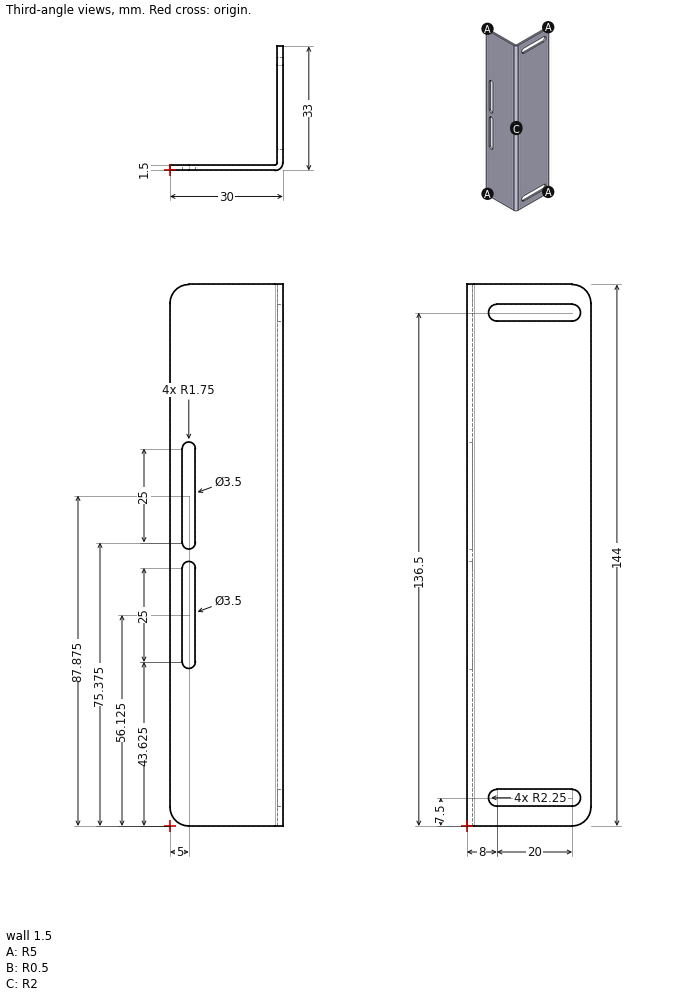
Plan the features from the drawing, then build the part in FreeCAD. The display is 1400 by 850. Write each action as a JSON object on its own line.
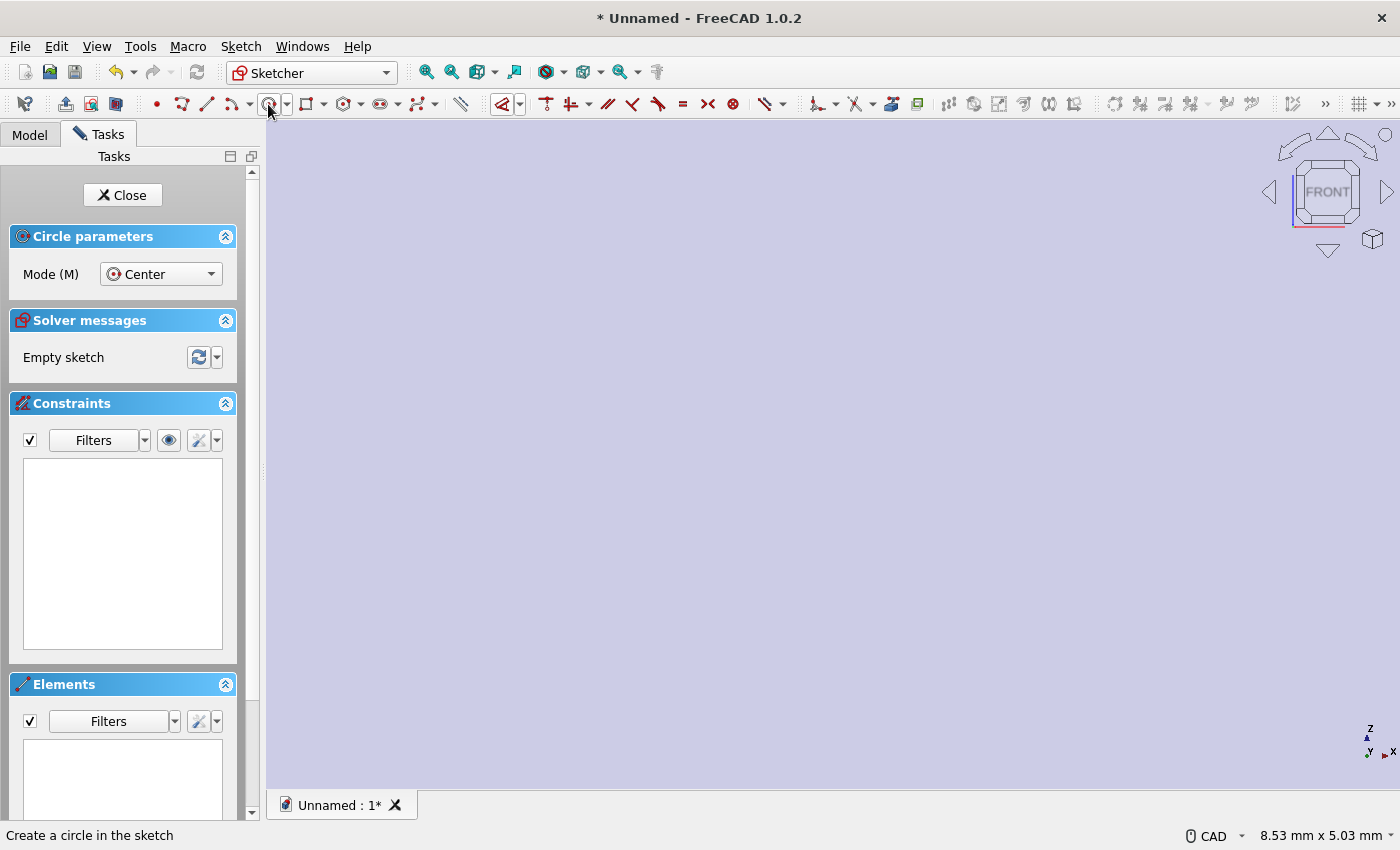
{"action": "left_click", "coordinate": [764, 454]}
{"action": "left_click", "coordinate": [929, 290]}
{"action": "key", "text": "Escape"}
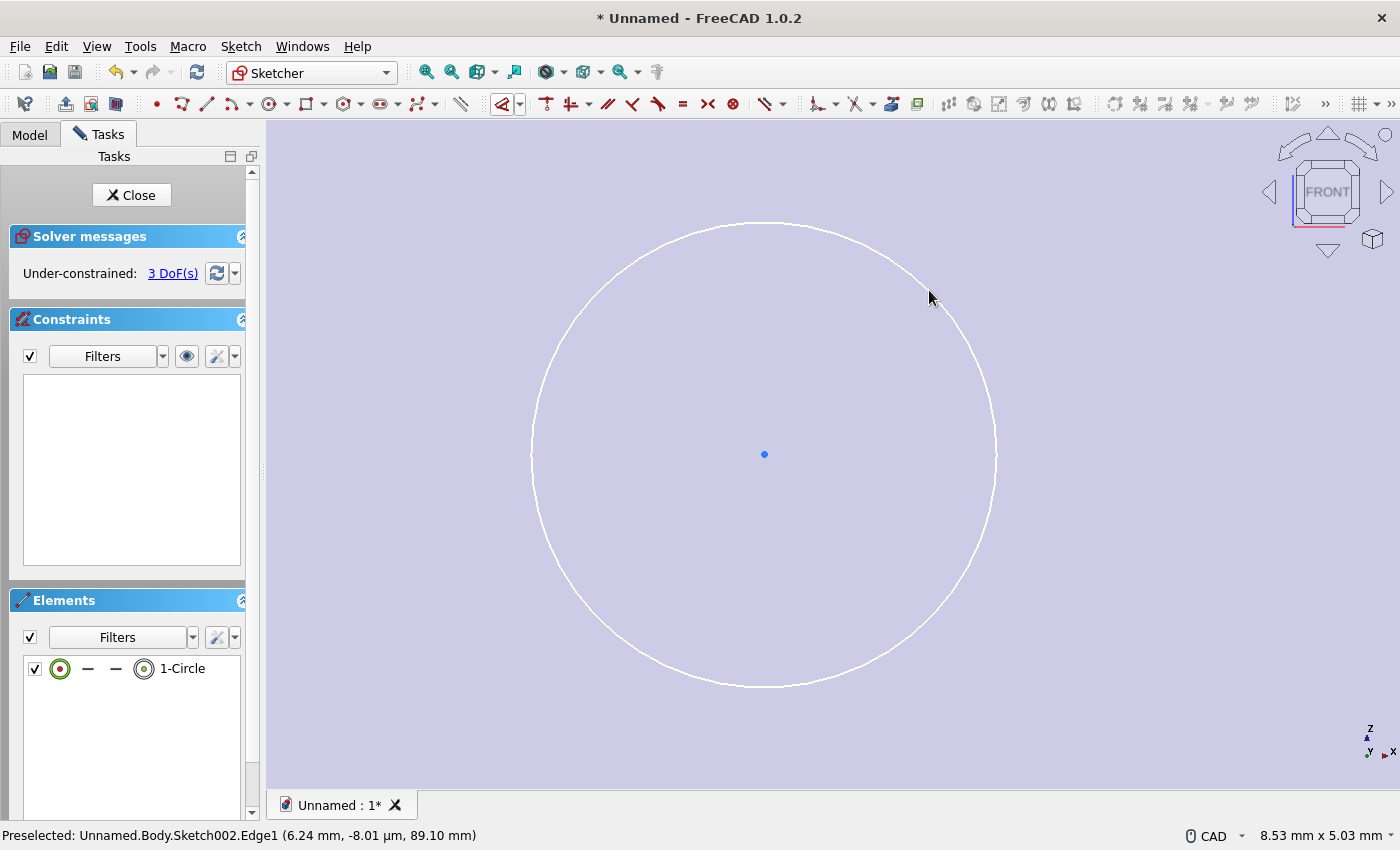
{"action": "left_click", "coordinate": [928, 290]}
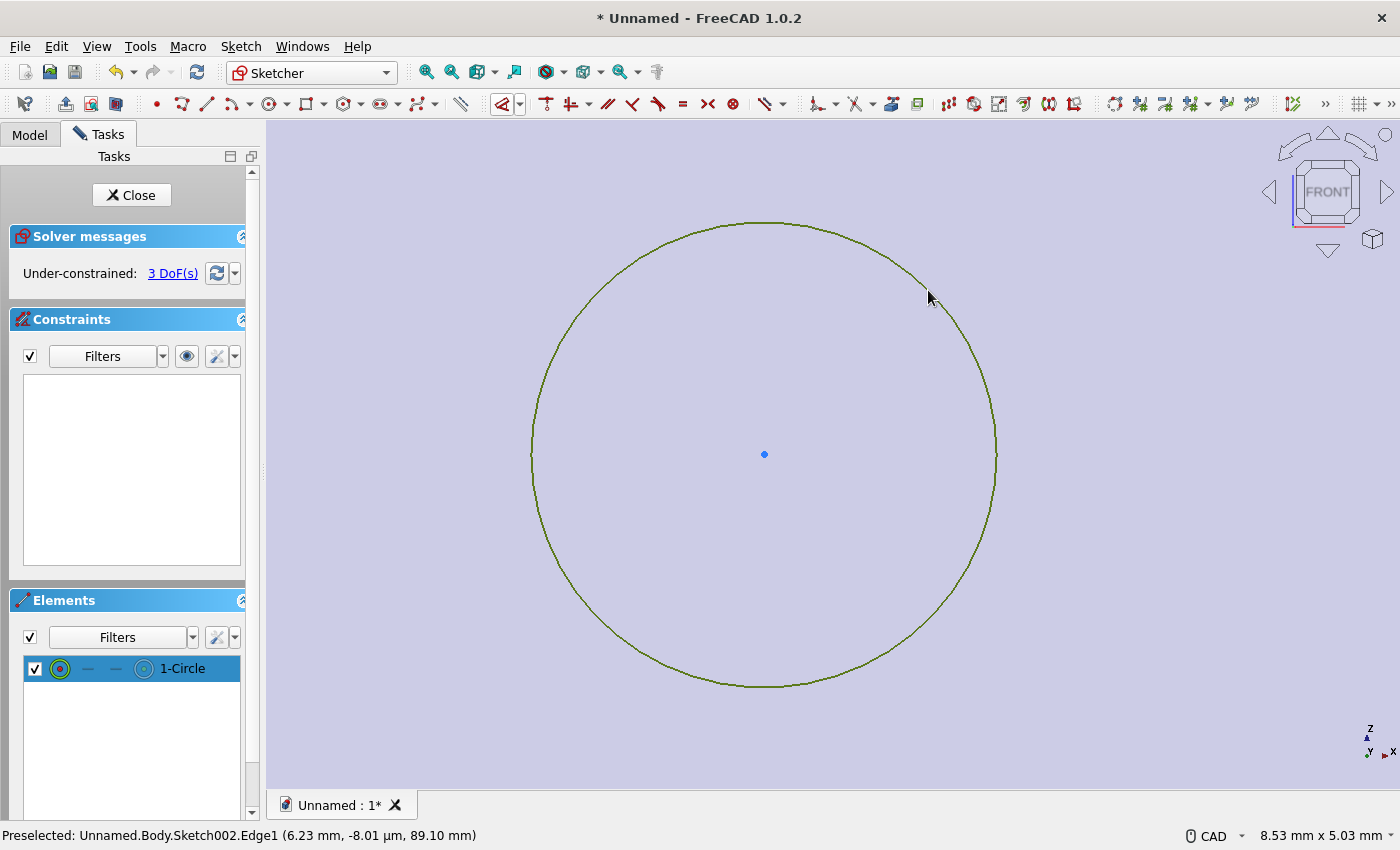
{"action": "key", "text": "k o"}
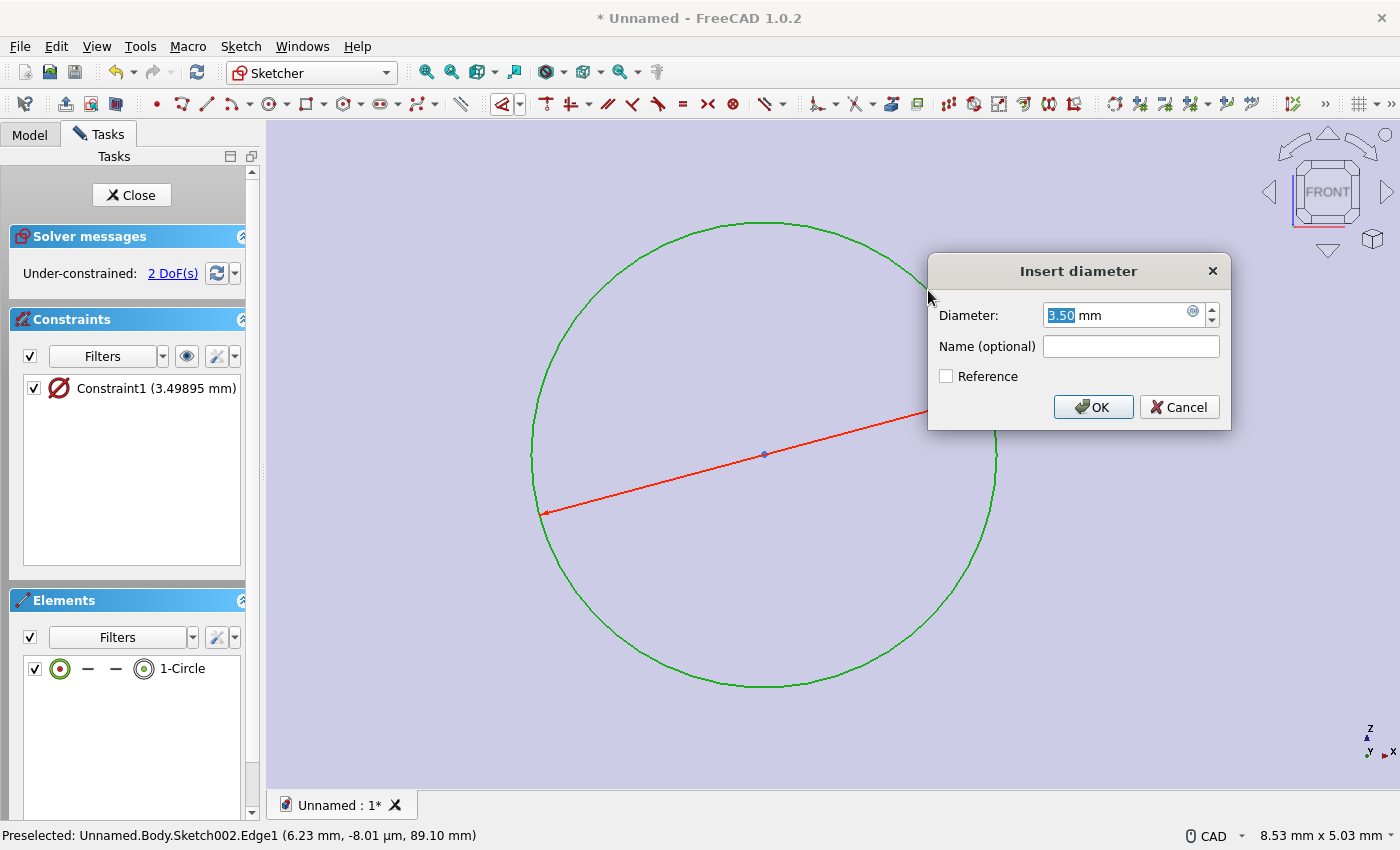
{"action": "type", "text": "3.5"}
{"action": "key", "text": "Return"}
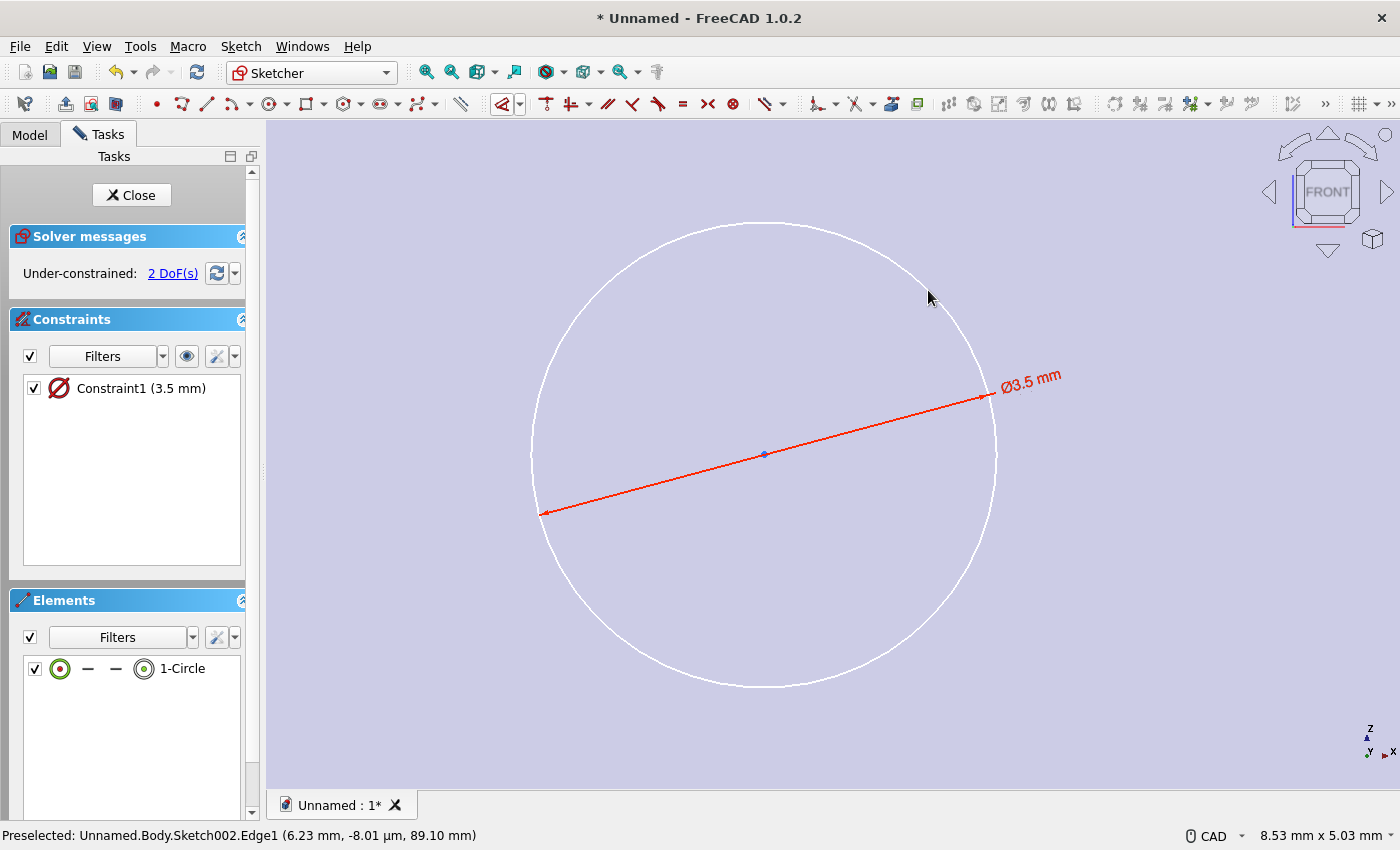
{"action": "left_click", "coordinate": [764, 455]}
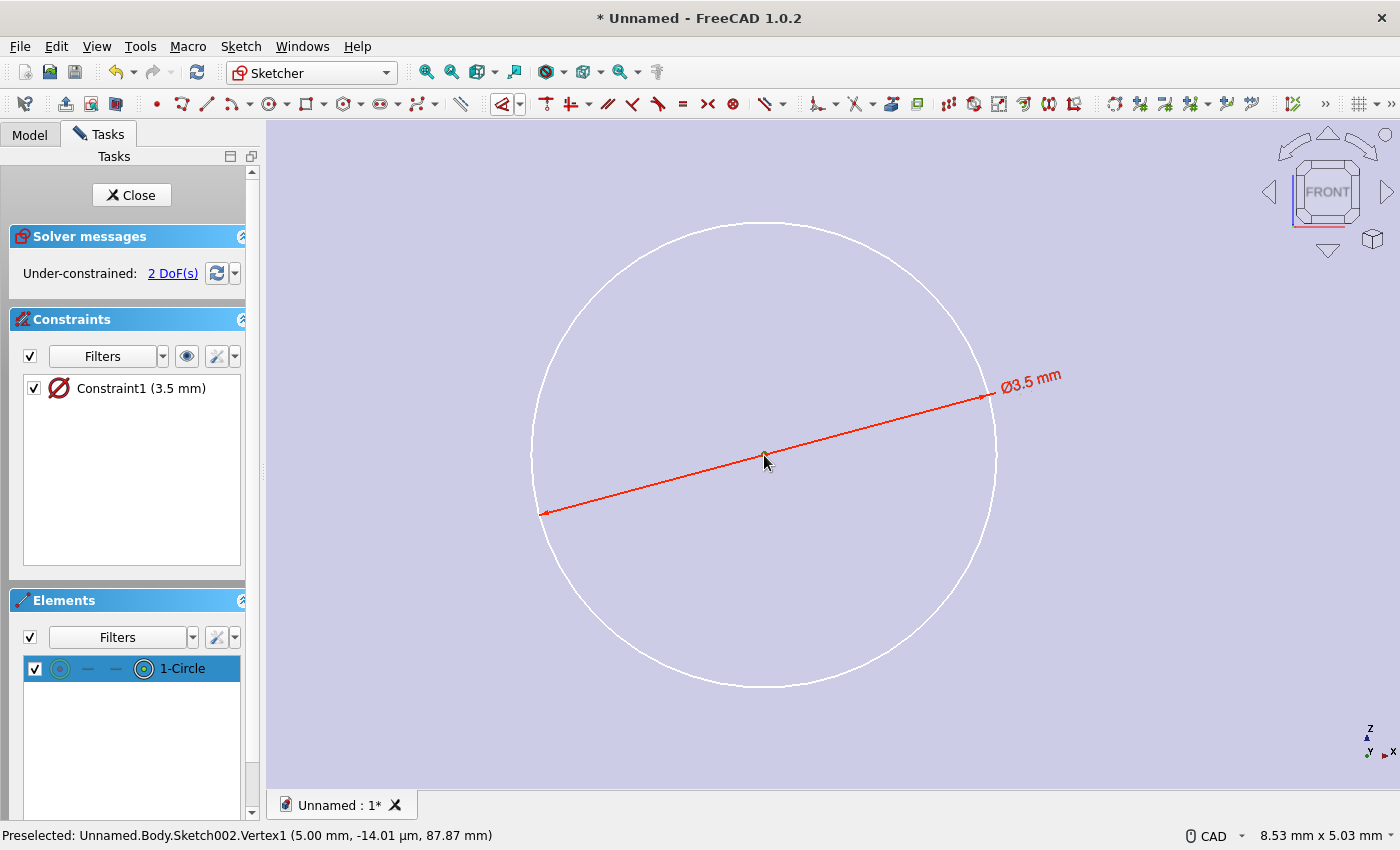
{"action": "left_click", "coordinate": [520, 104]}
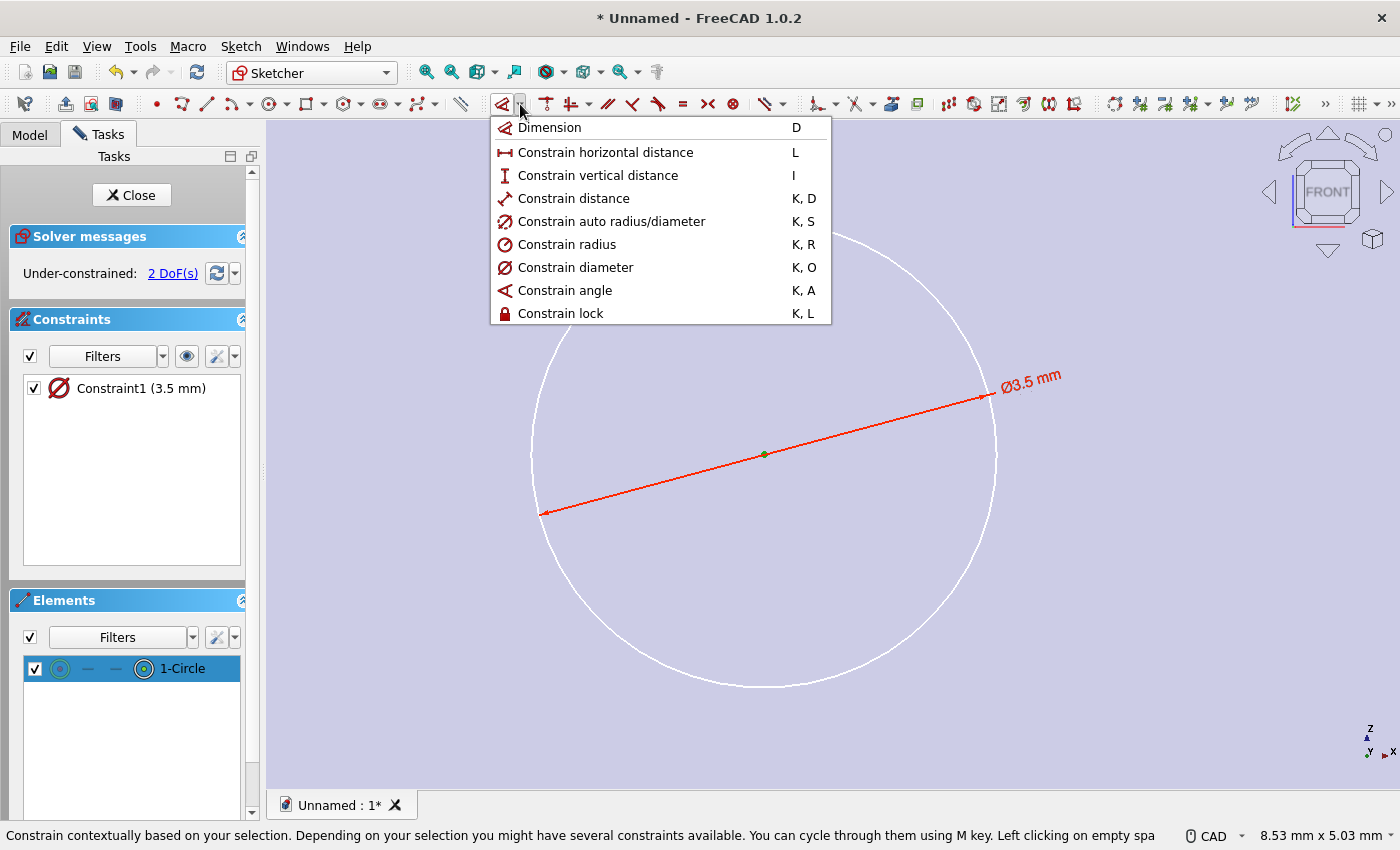
{"action": "left_click", "coordinate": [661, 152]}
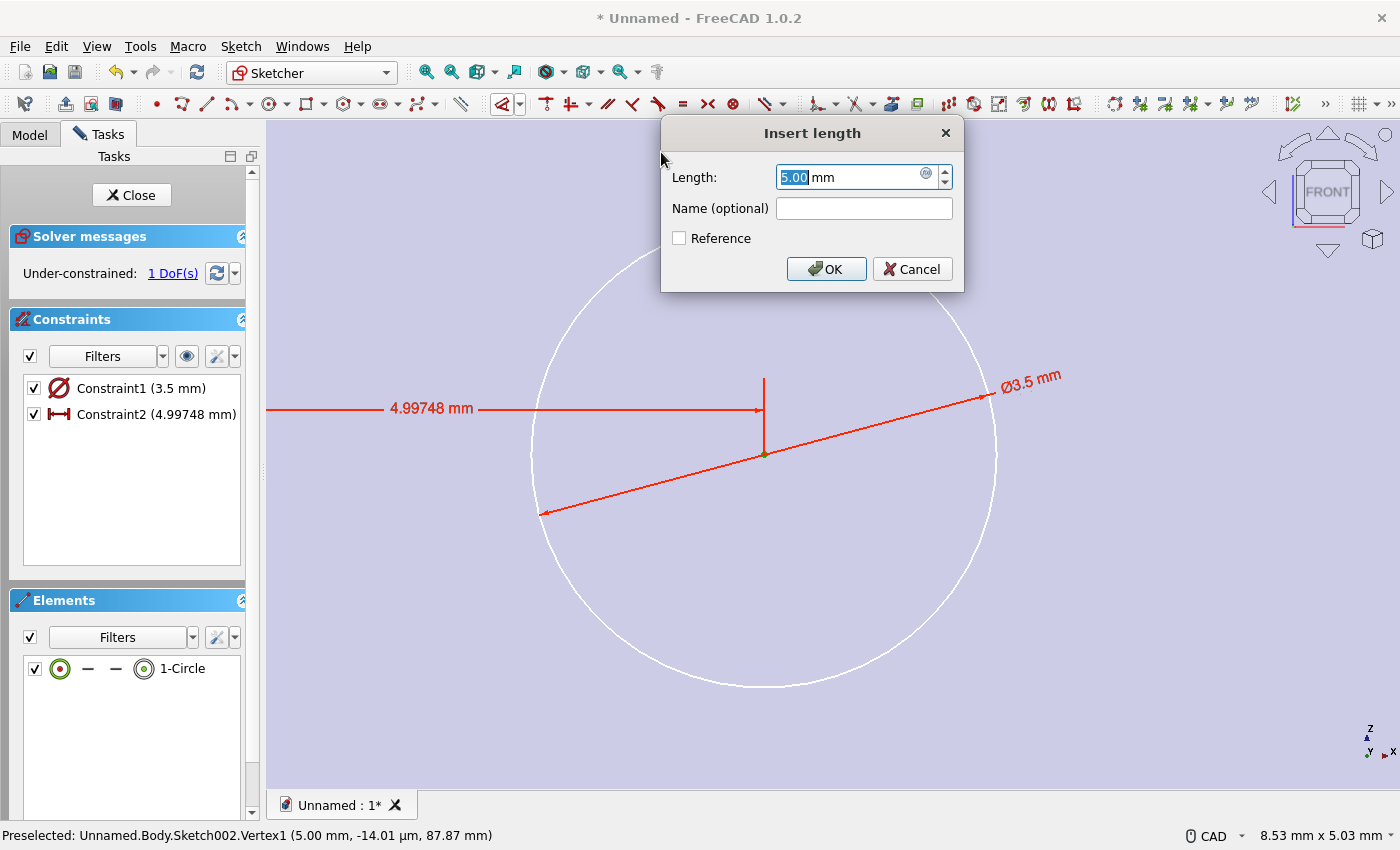
{"action": "type", "text": "5"}
{"action": "key", "text": "Return"}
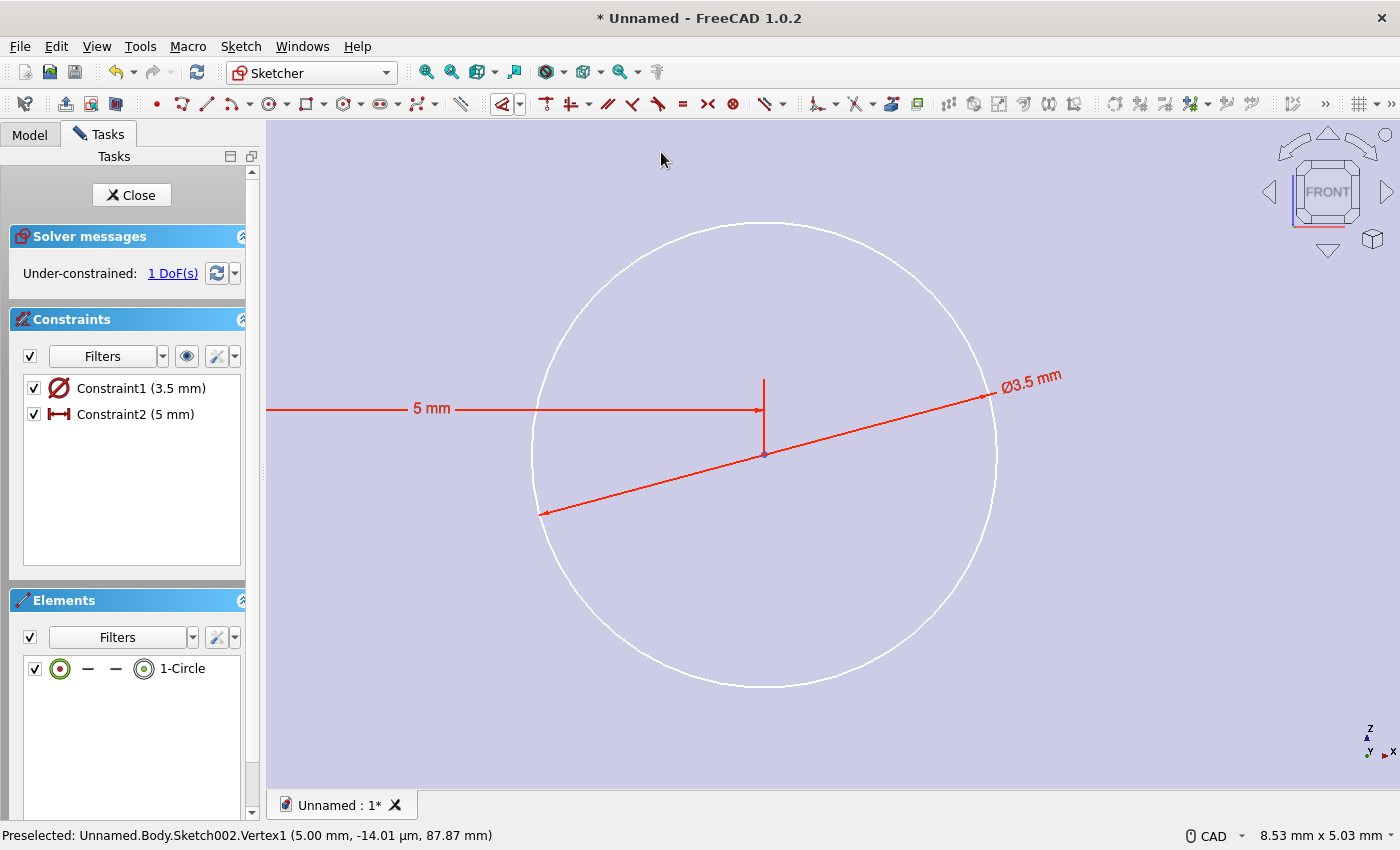
{"action": "left_click", "coordinate": [764, 455]}